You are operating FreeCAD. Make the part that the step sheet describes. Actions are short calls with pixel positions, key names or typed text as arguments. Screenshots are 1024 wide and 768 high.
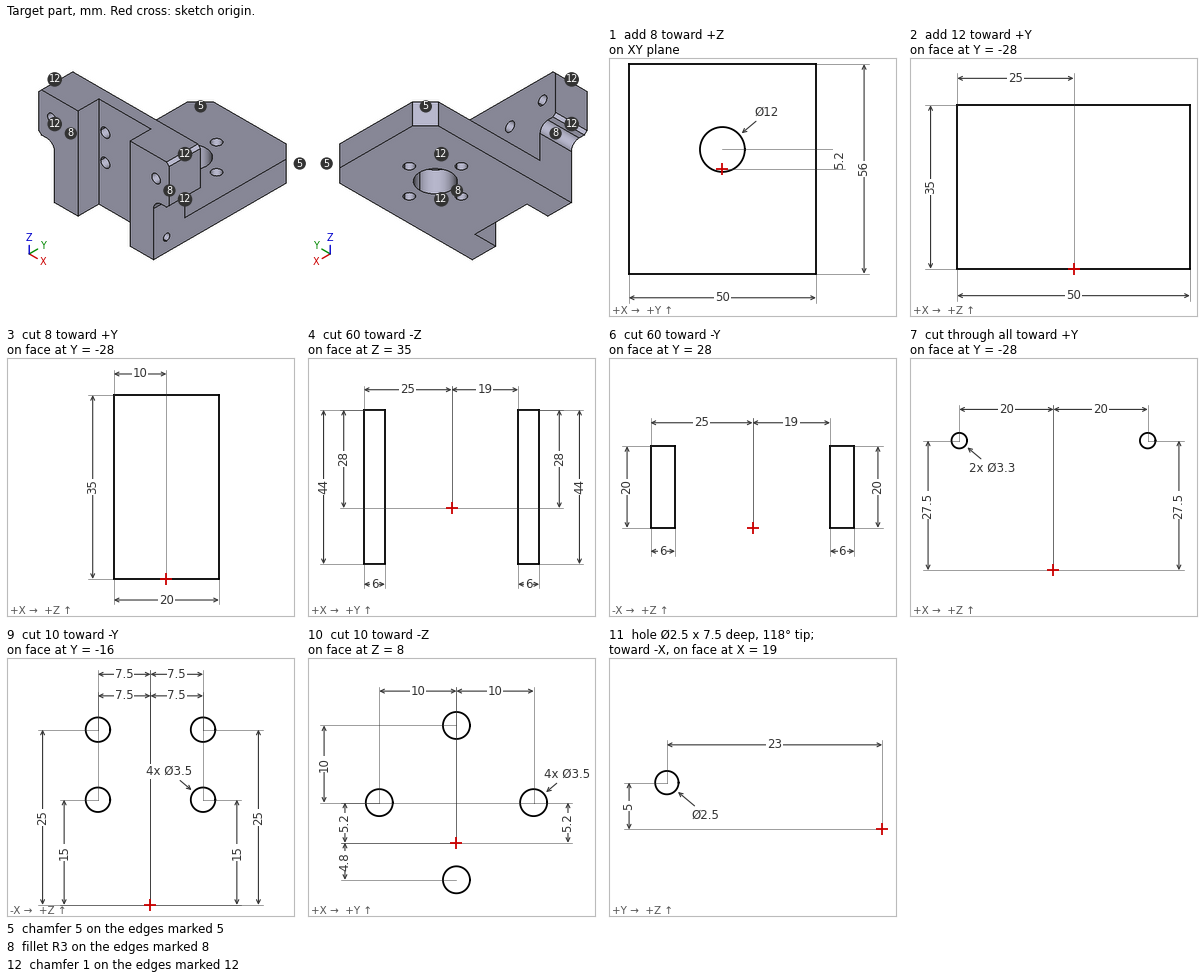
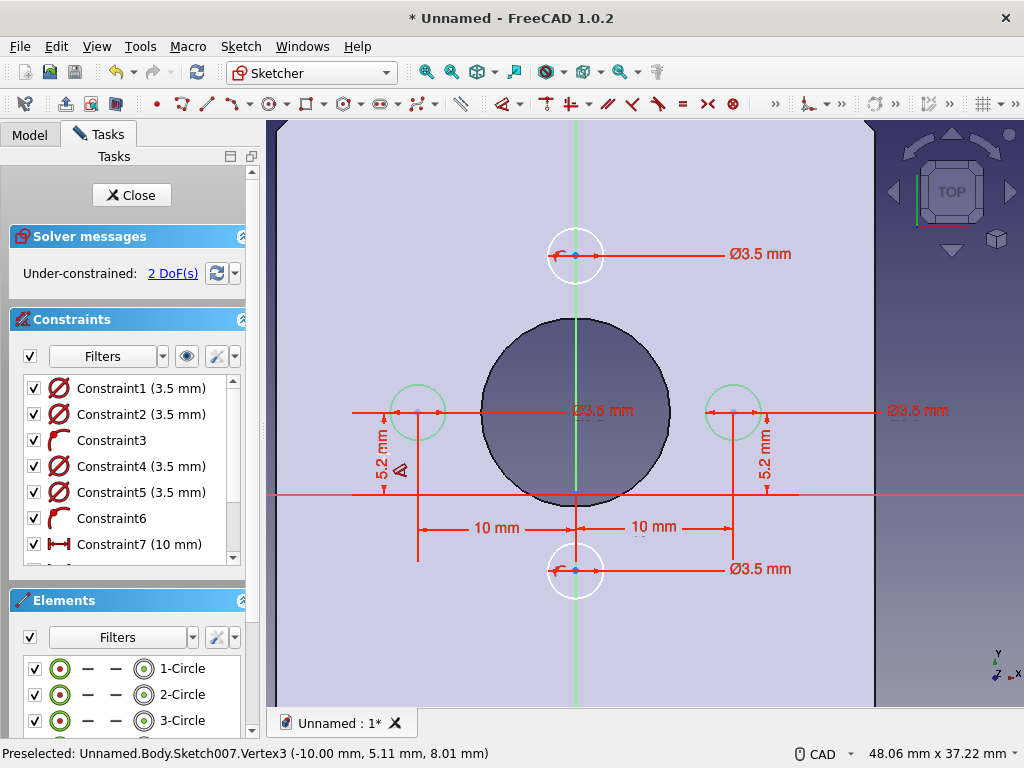
click(576, 571)
click(634, 550)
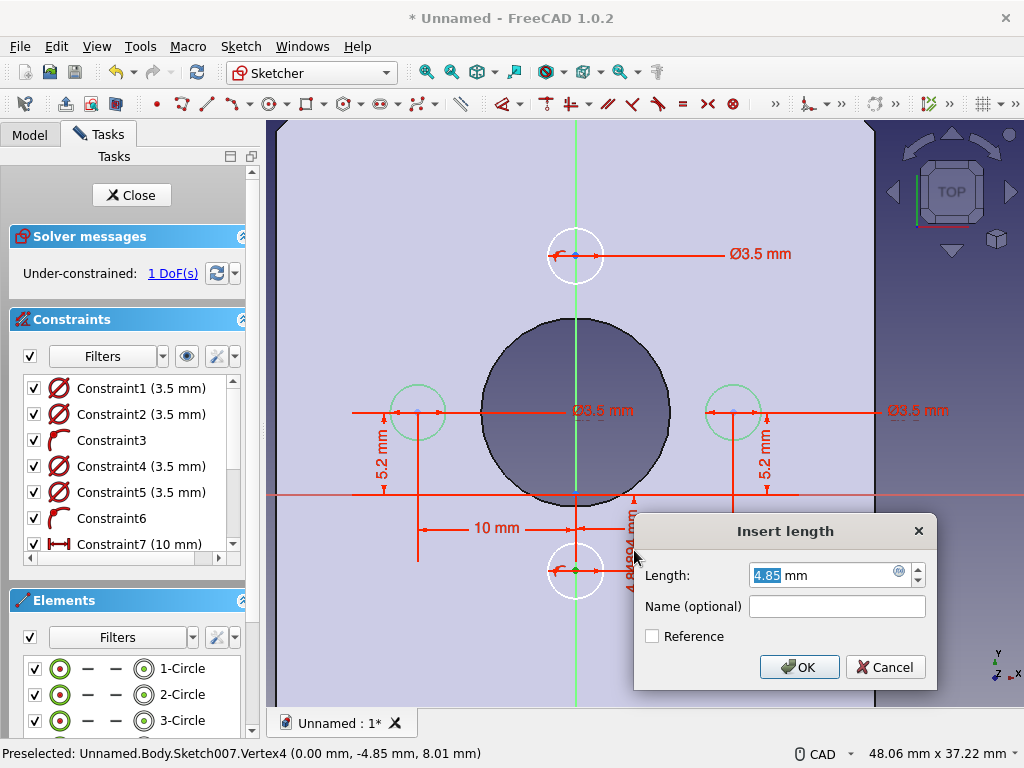
text(4.8)
key(Return)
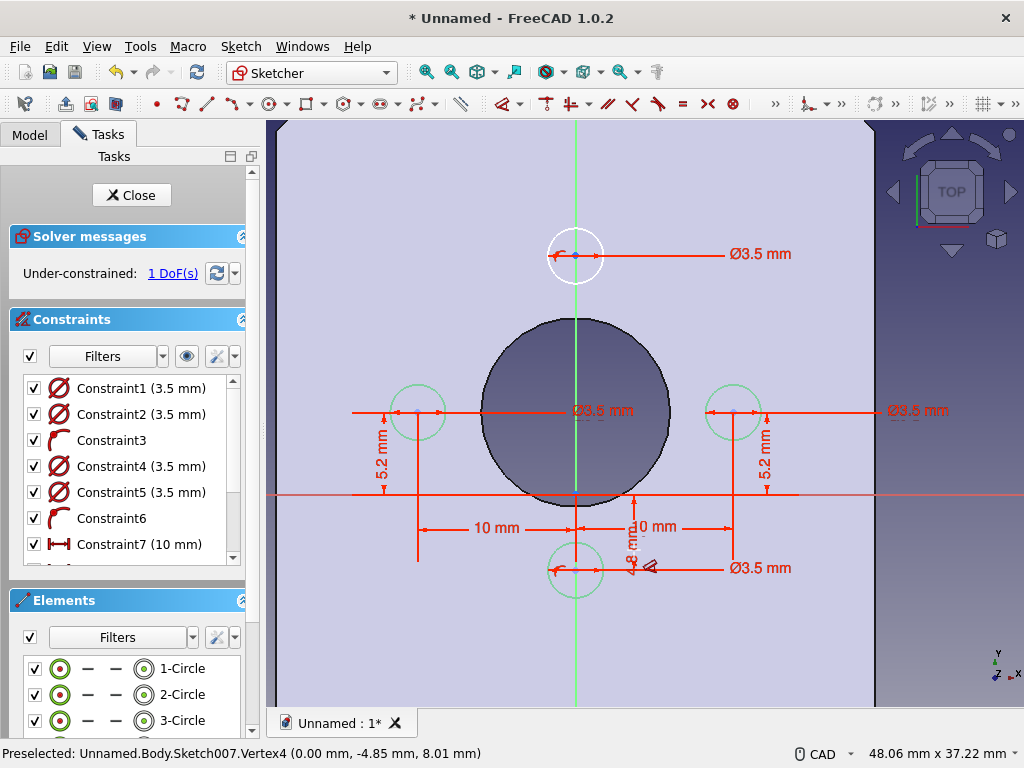
click(733, 413)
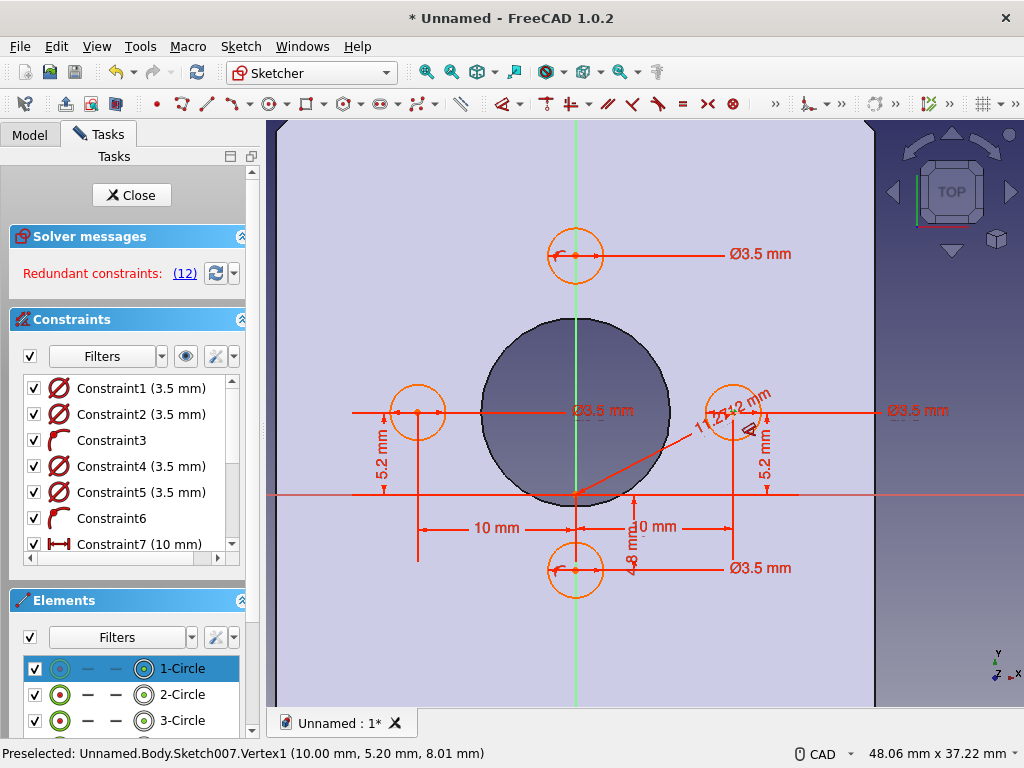
click(576, 256)
click(767, 334)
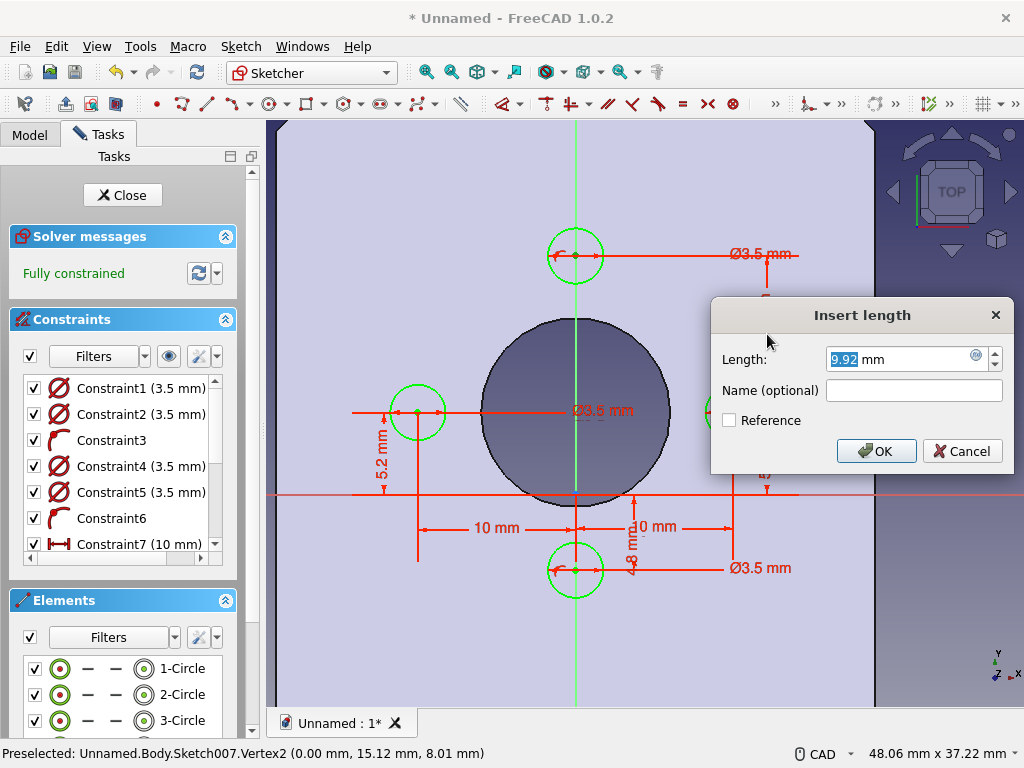
text(10)
key(Return)
key(Escape)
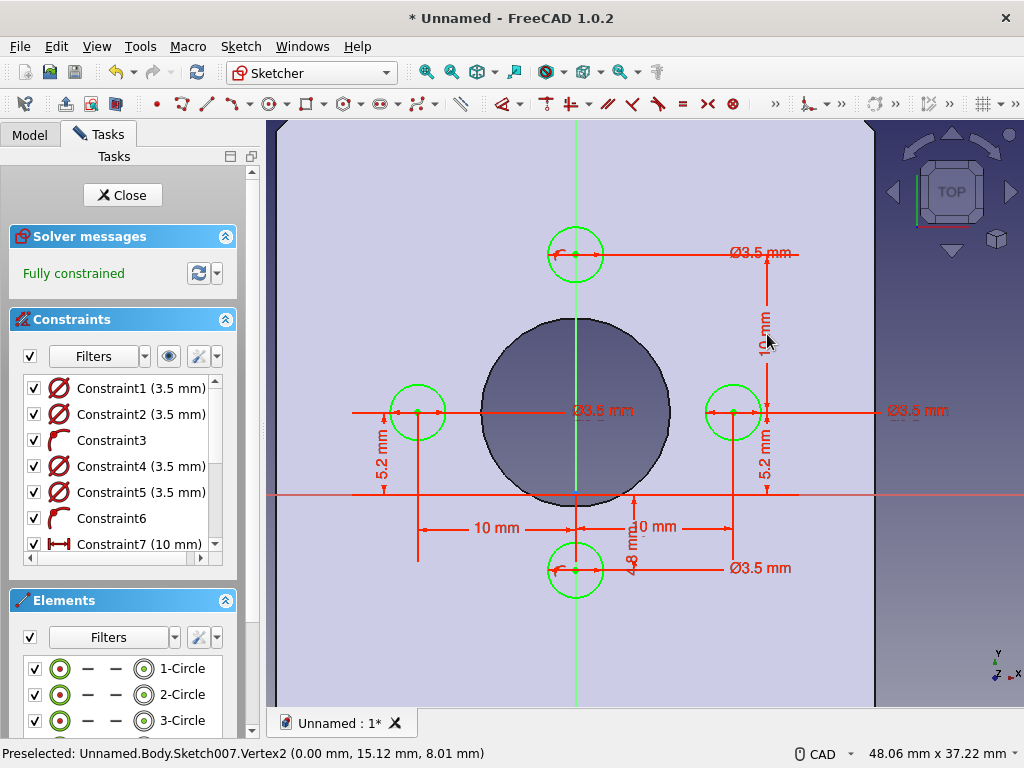
click(123, 195)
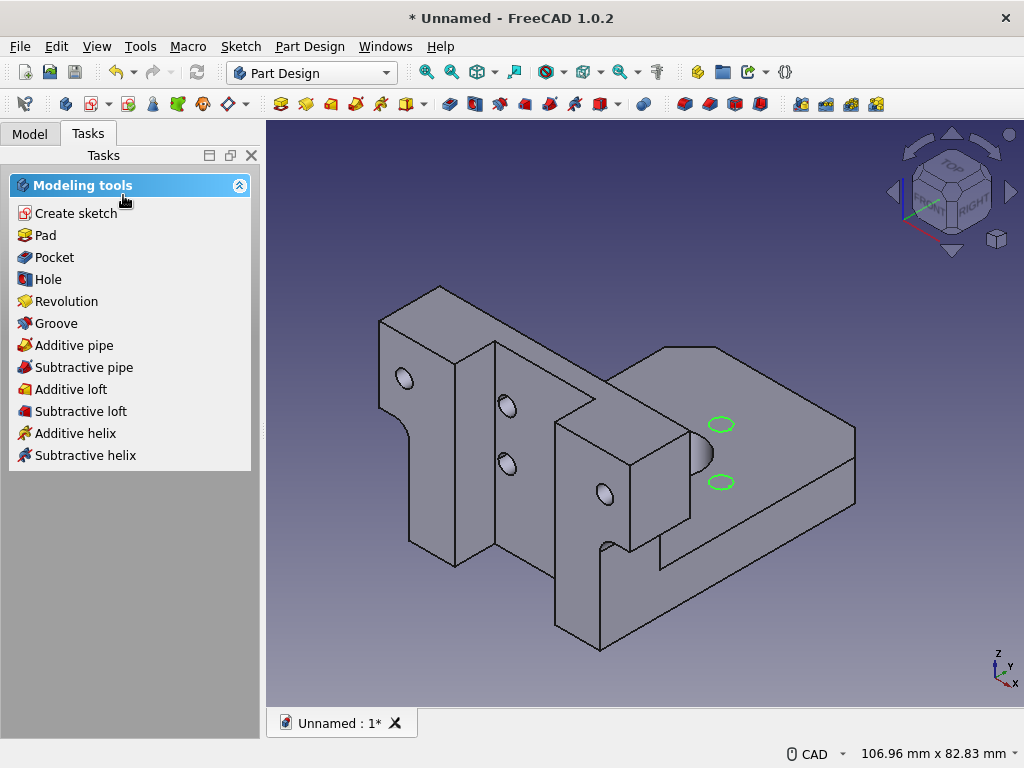
click(450, 104)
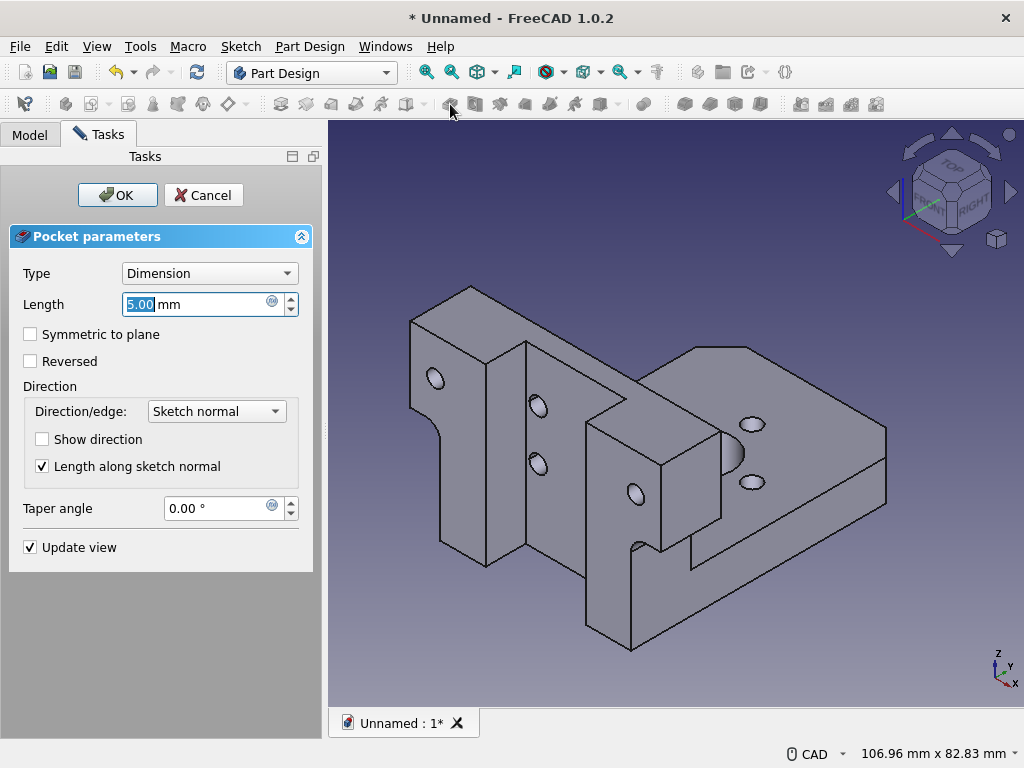
text(10)
key(Tab)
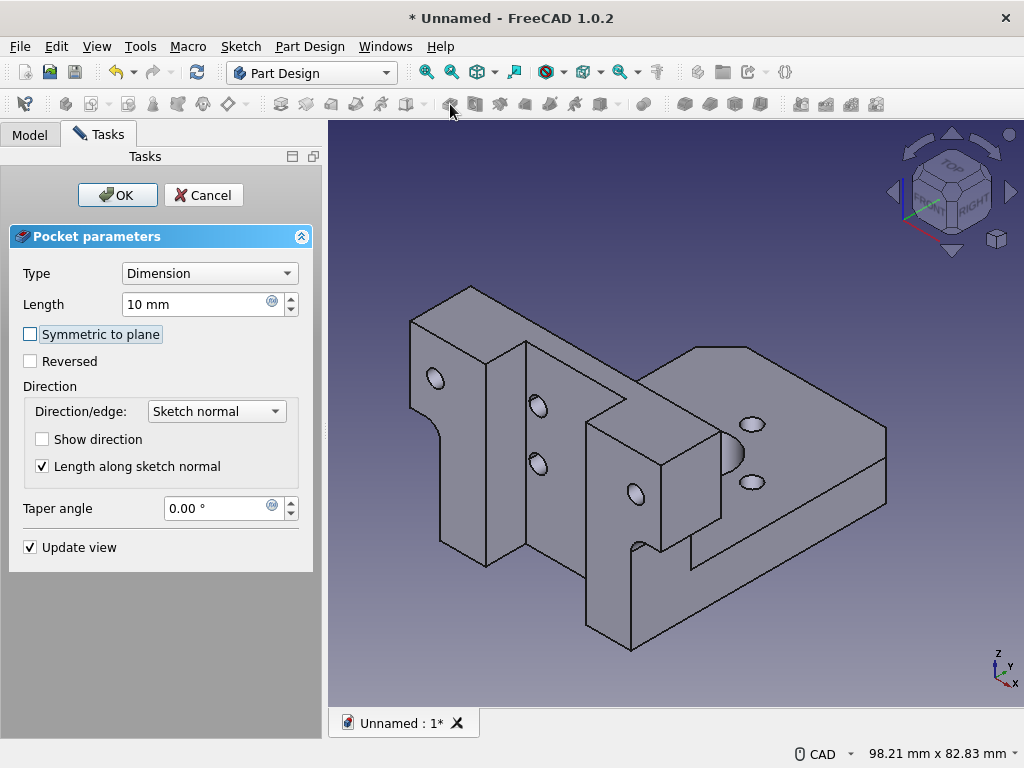
click(118, 195)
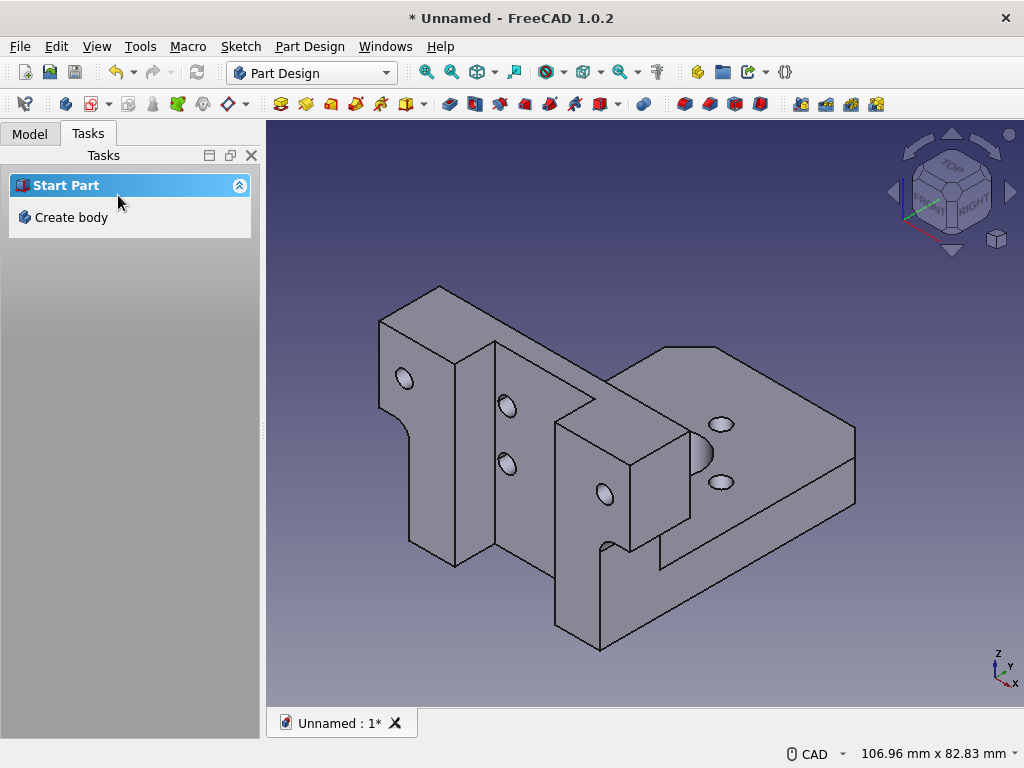
click(801, 513)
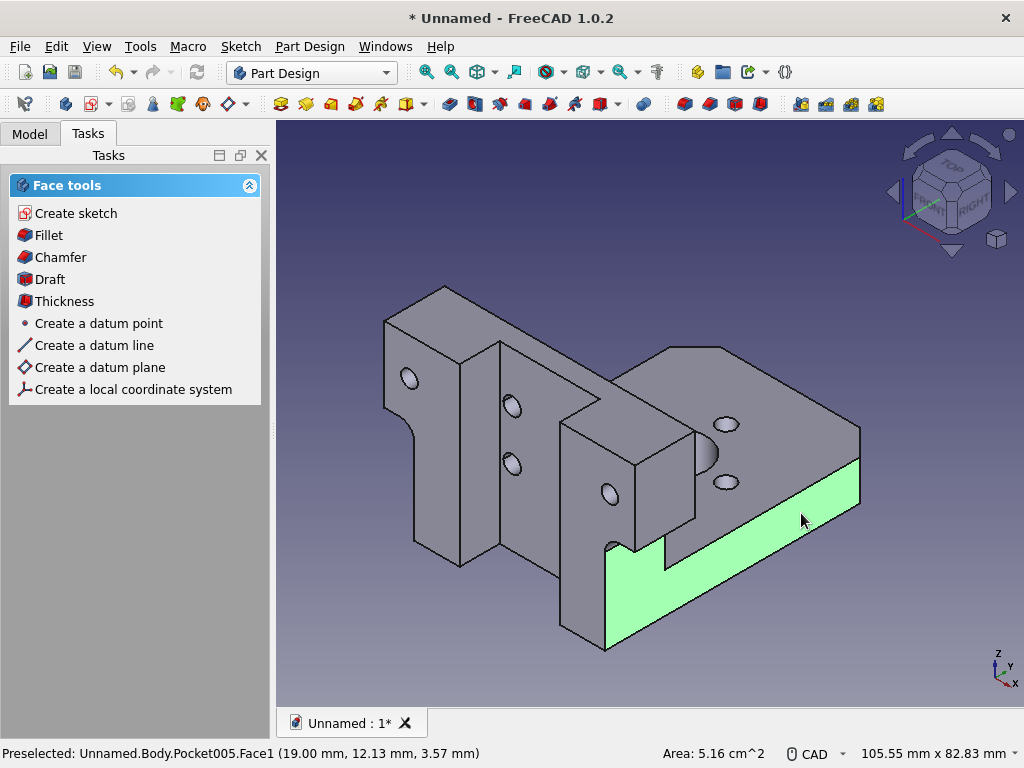
click(90, 104)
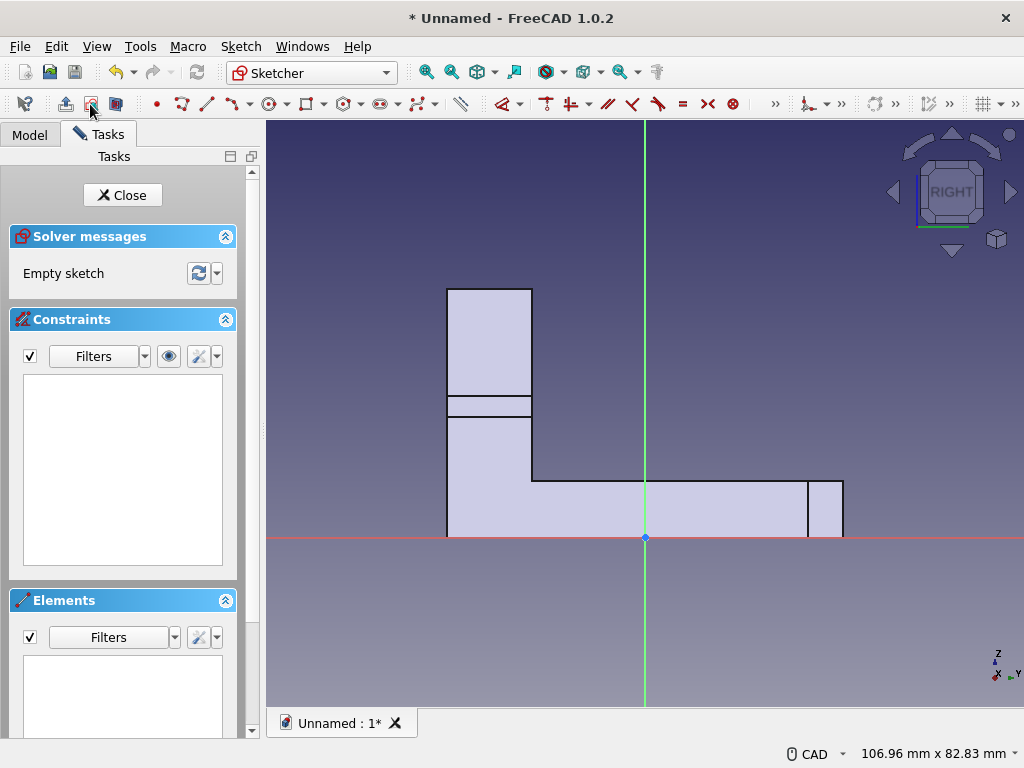
scroll(477, 507, up, 15)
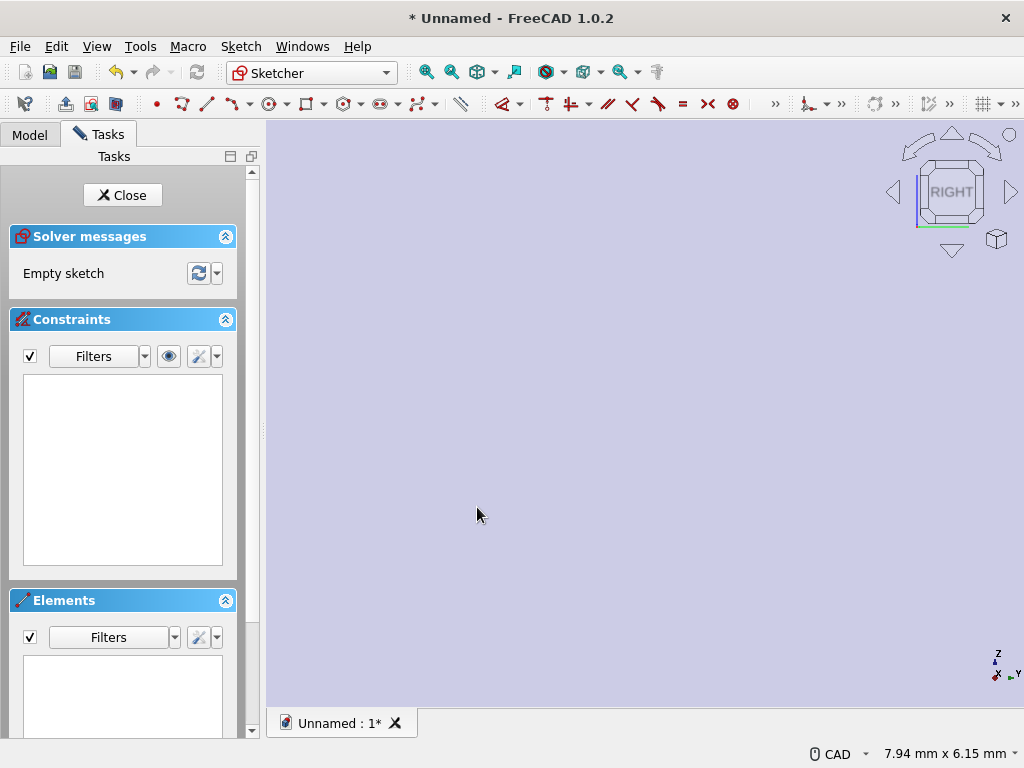
click(268, 104)